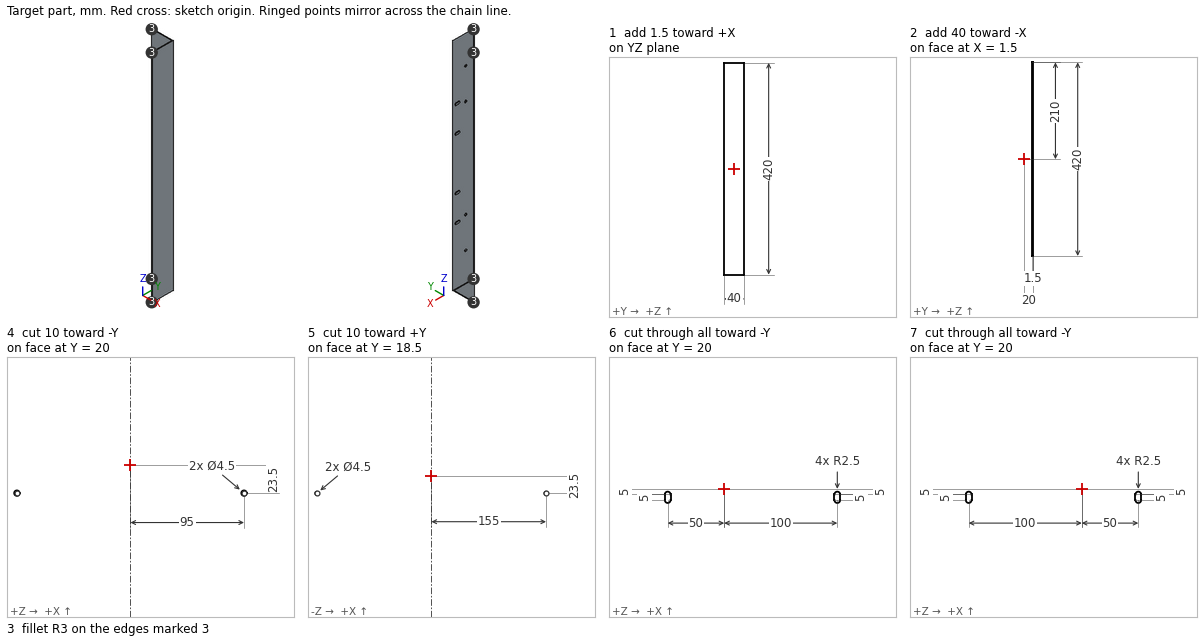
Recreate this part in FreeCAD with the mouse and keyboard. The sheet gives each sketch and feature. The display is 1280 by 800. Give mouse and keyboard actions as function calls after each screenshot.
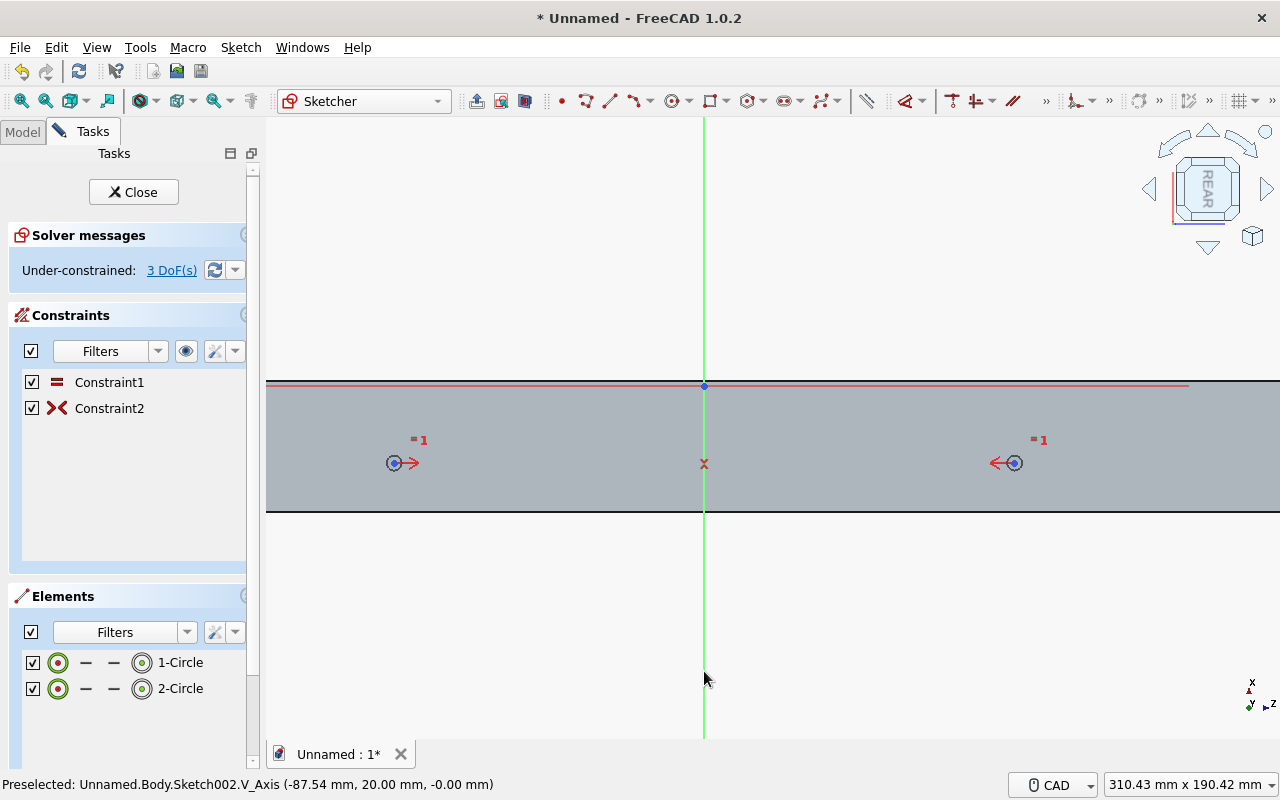
scroll(1020, 468, up, 5)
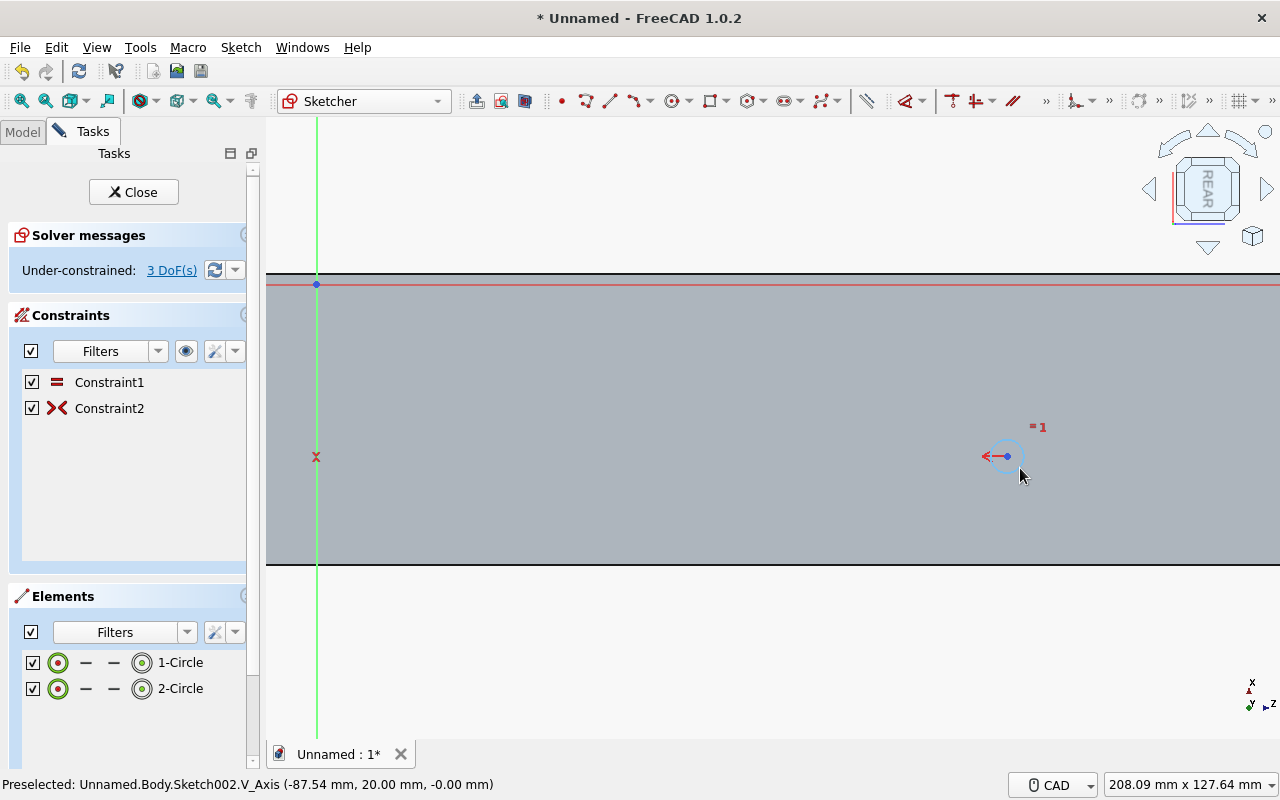
click(1018, 468)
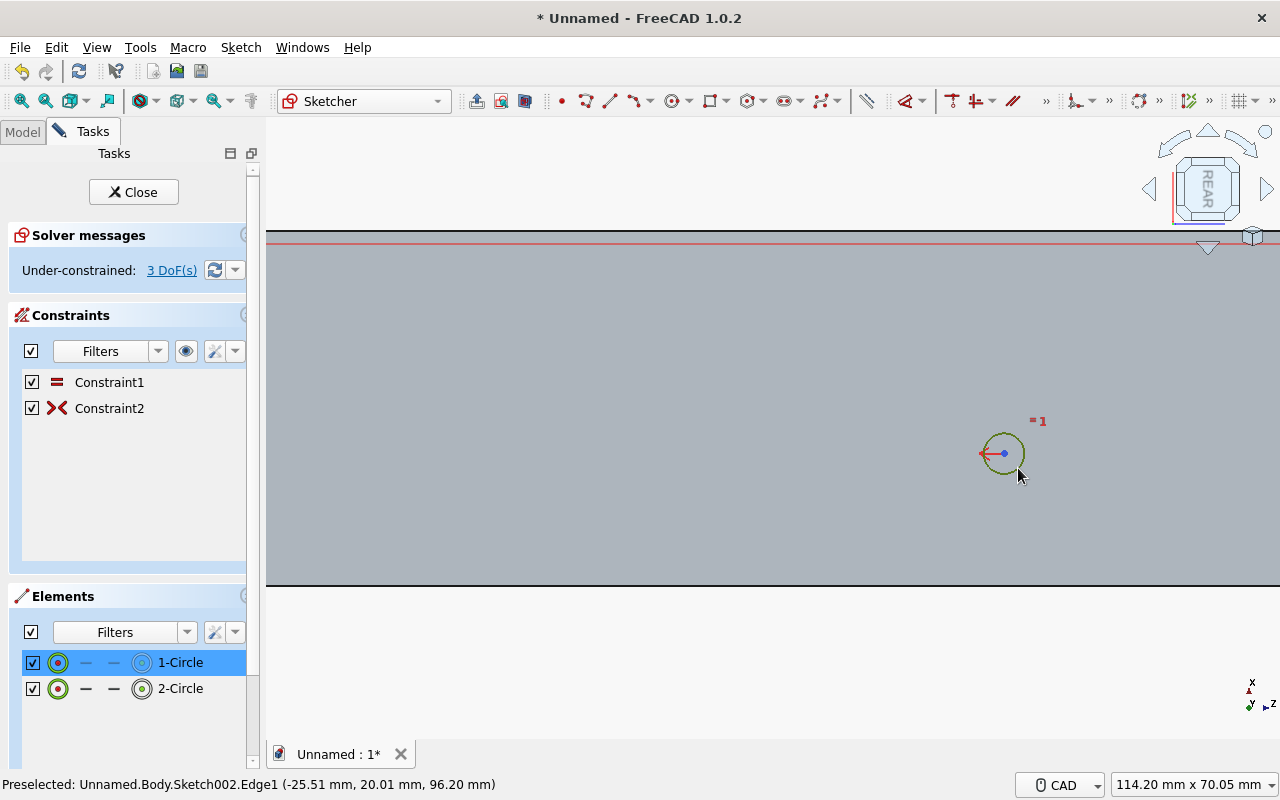
click(924, 102)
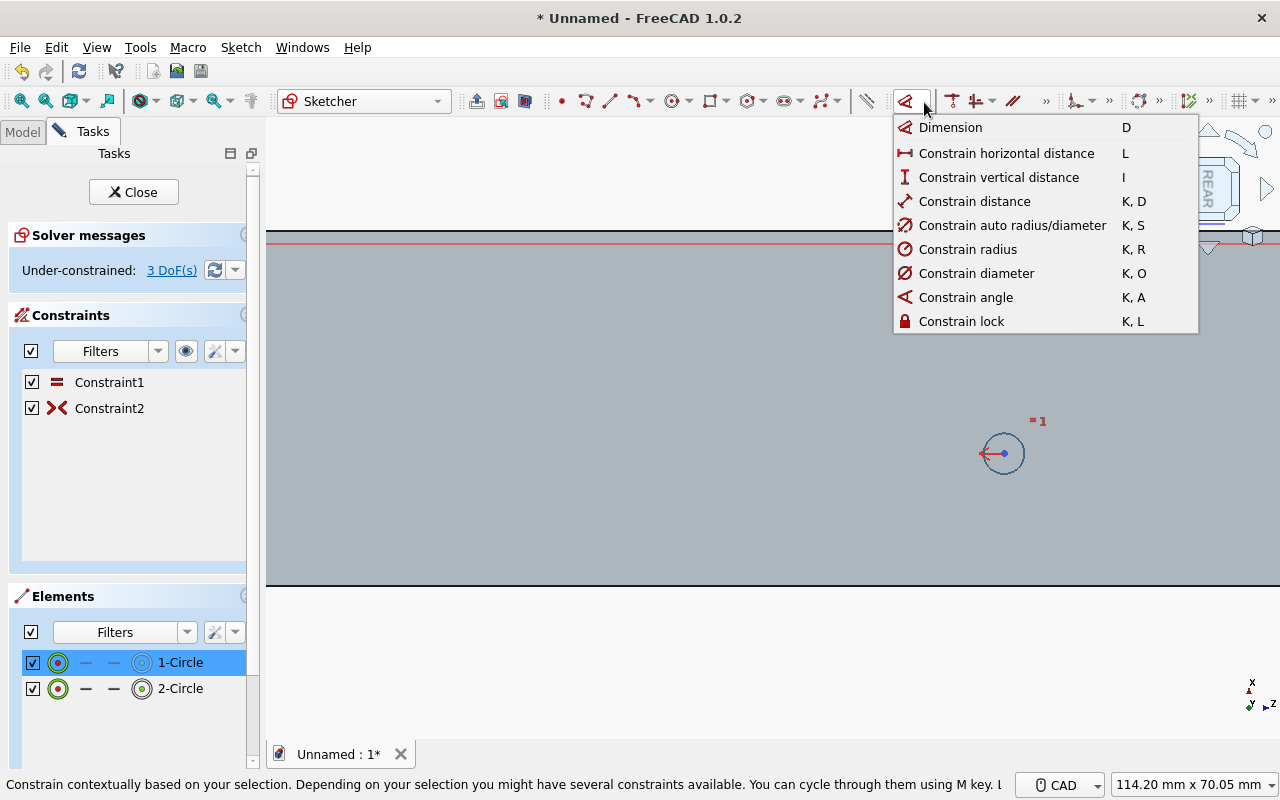
click(1046, 273)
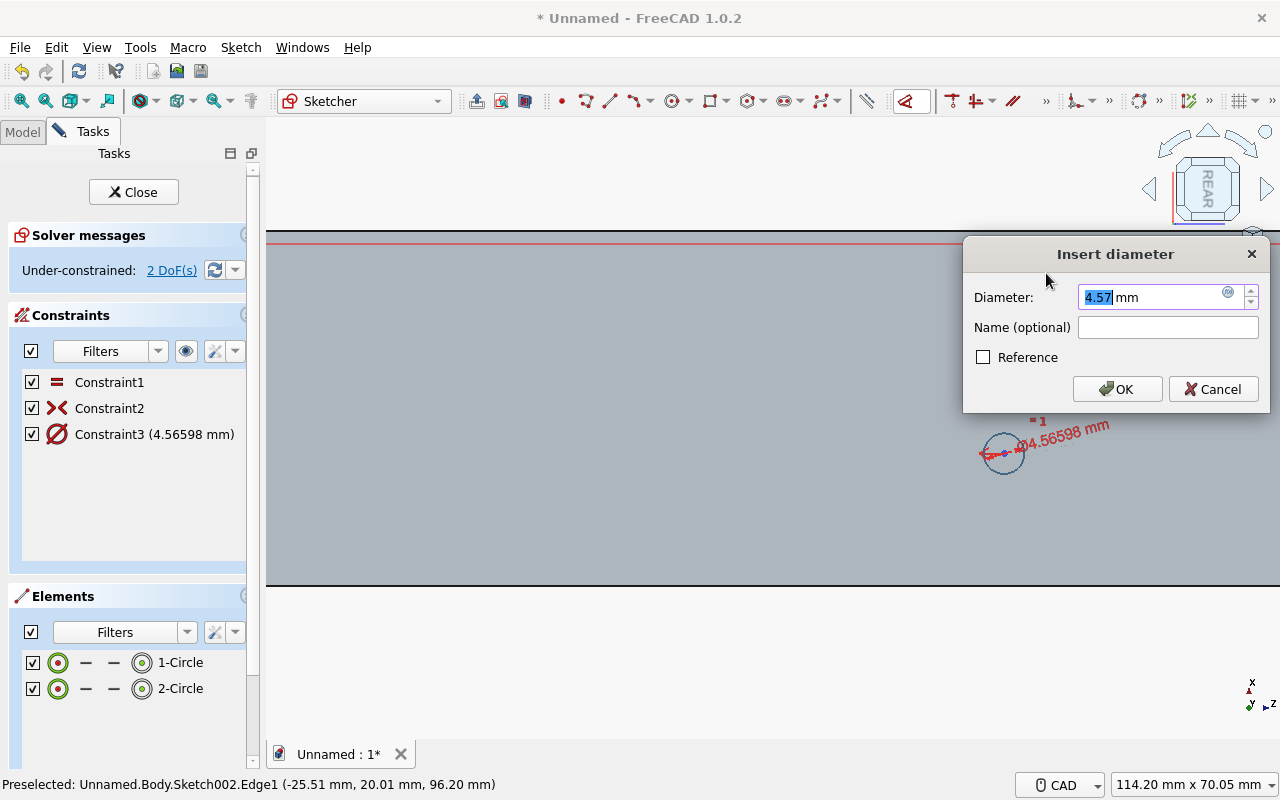
text(4.5)
key(Return)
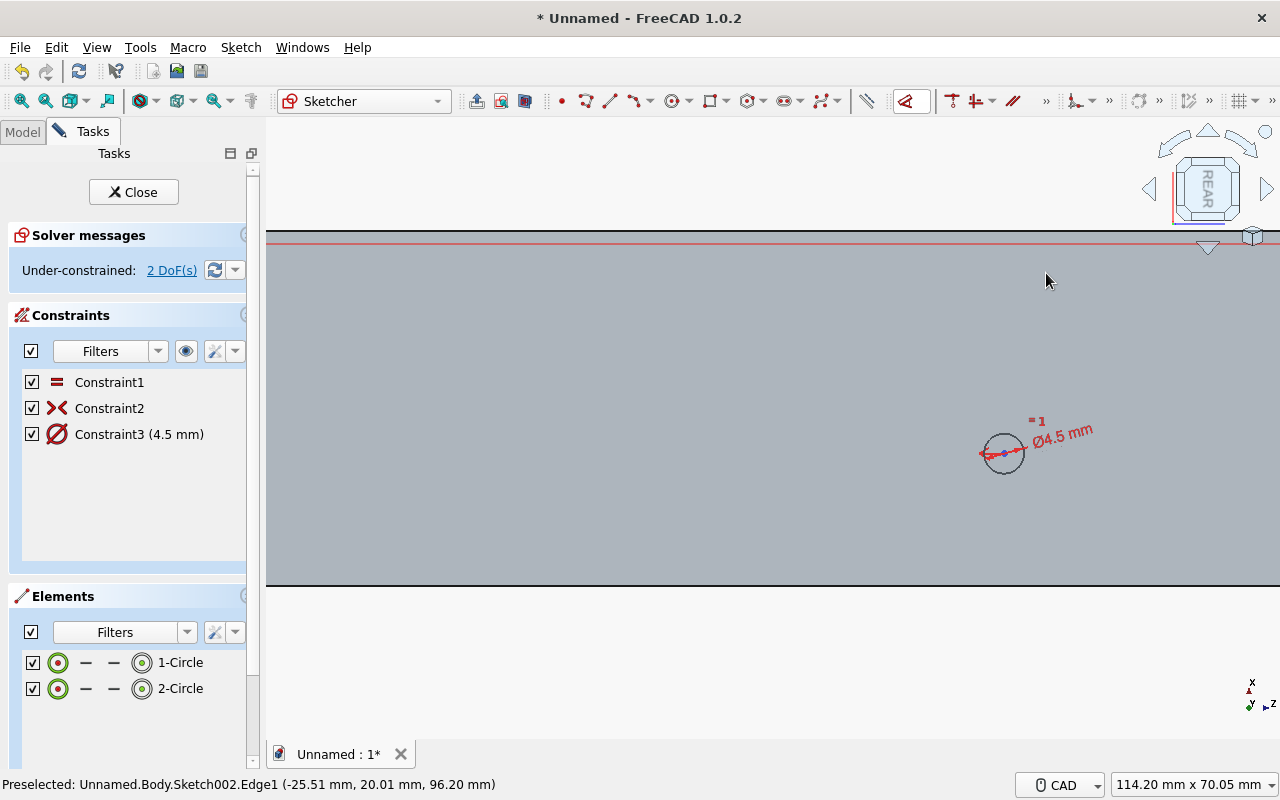
click(1004, 454)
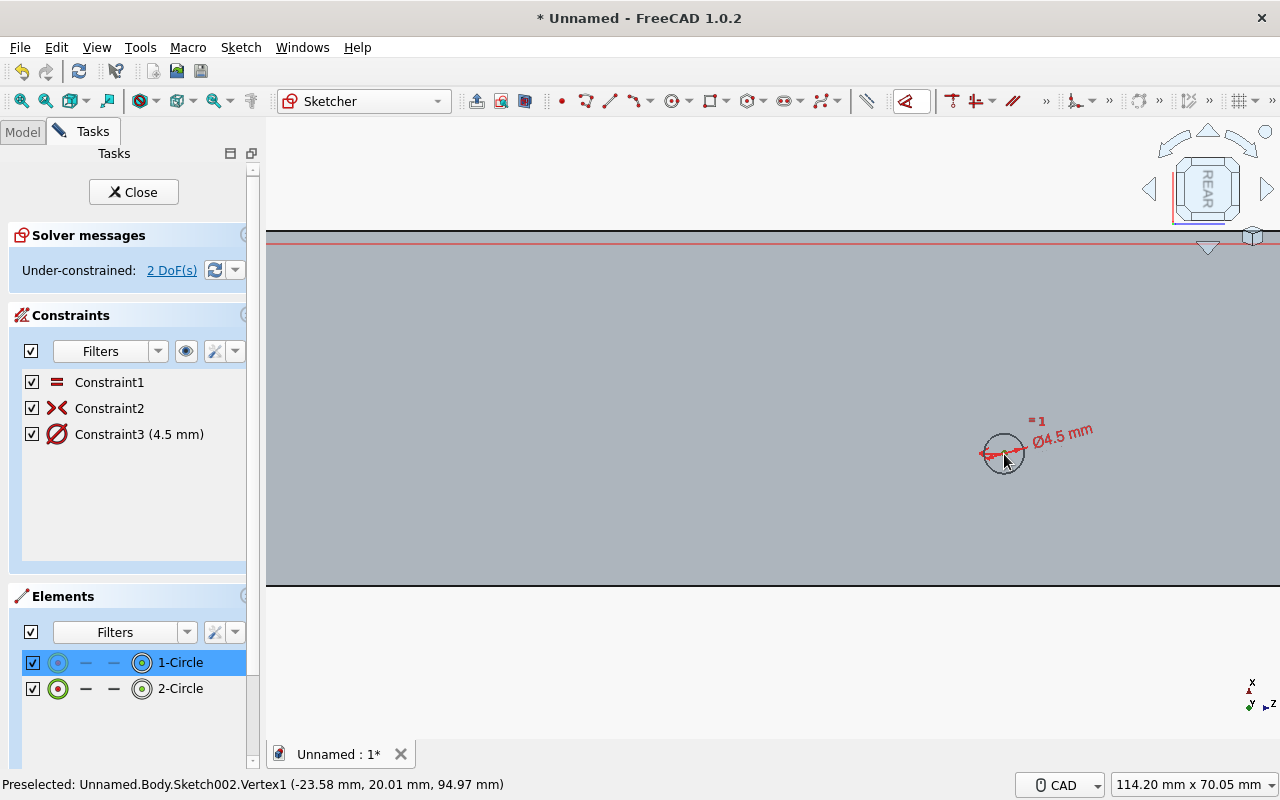
click(924, 102)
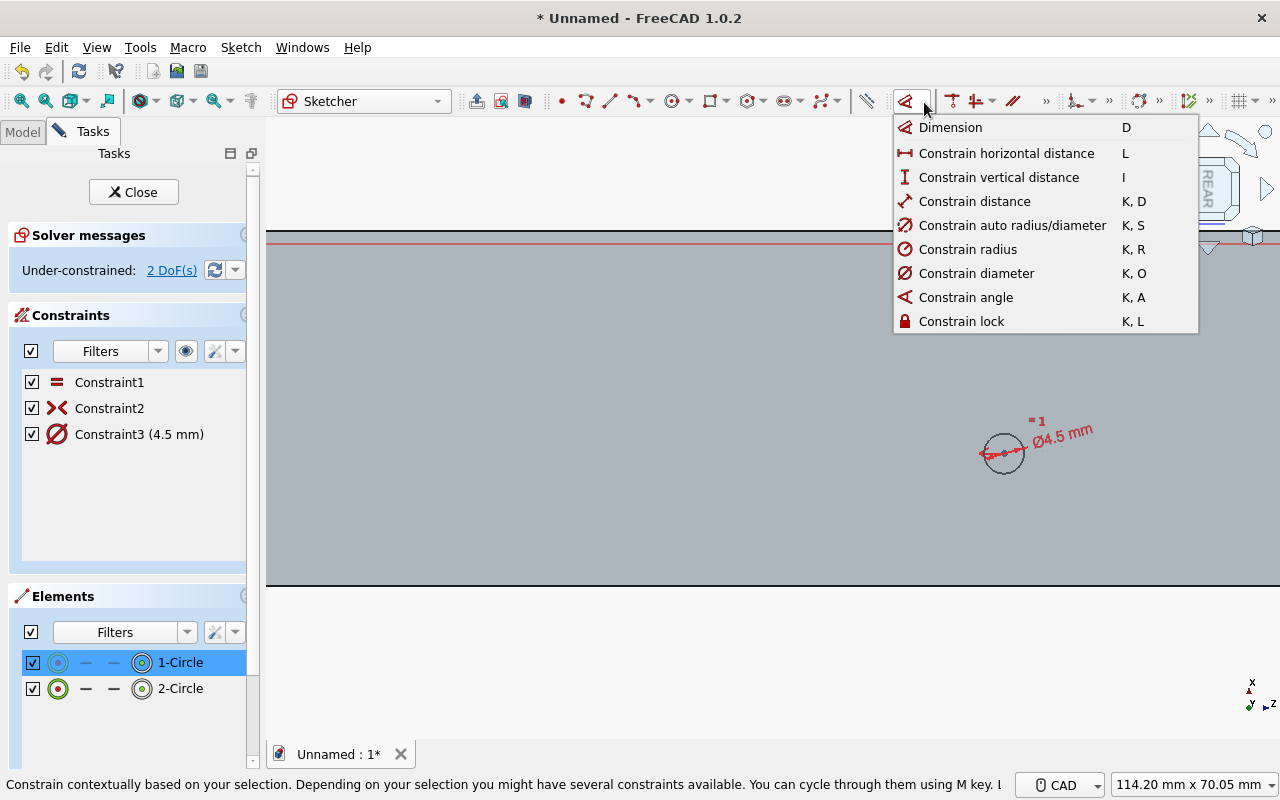
click(1046, 153)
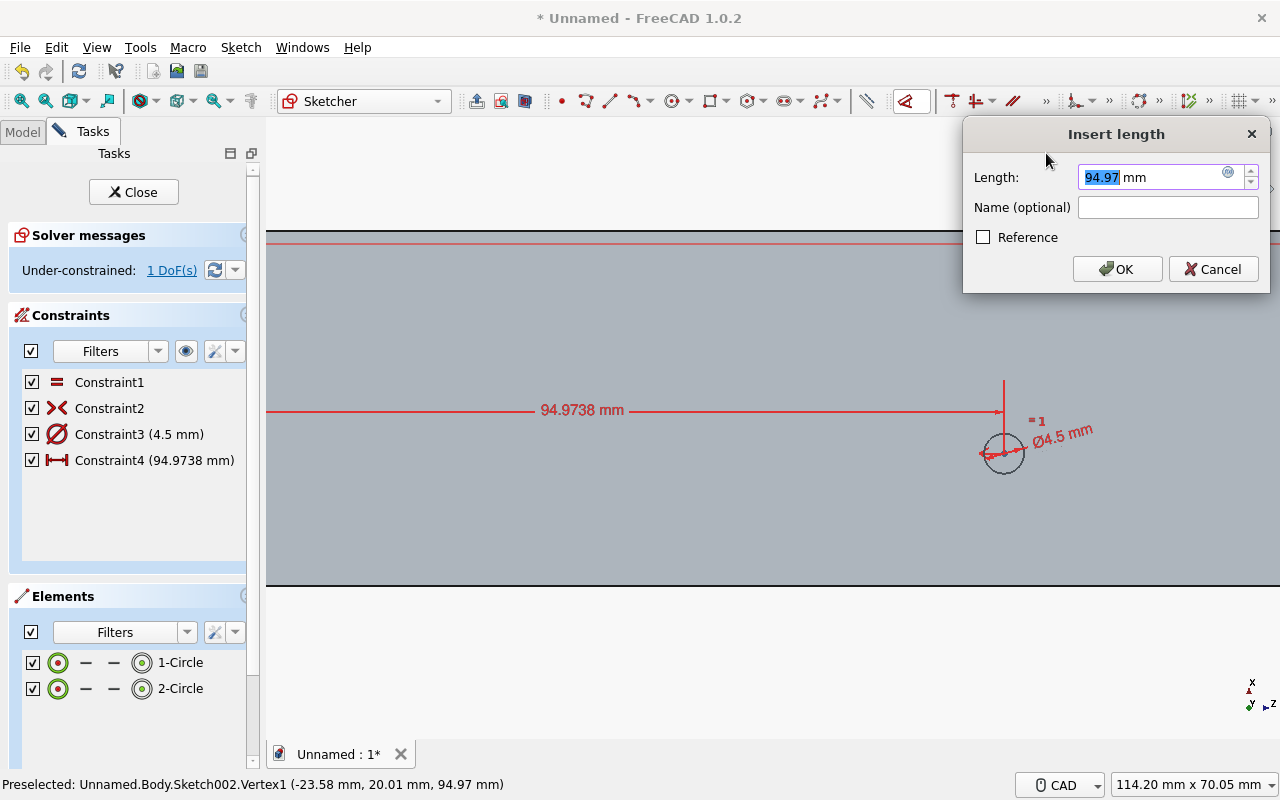
text(95)
key(Return)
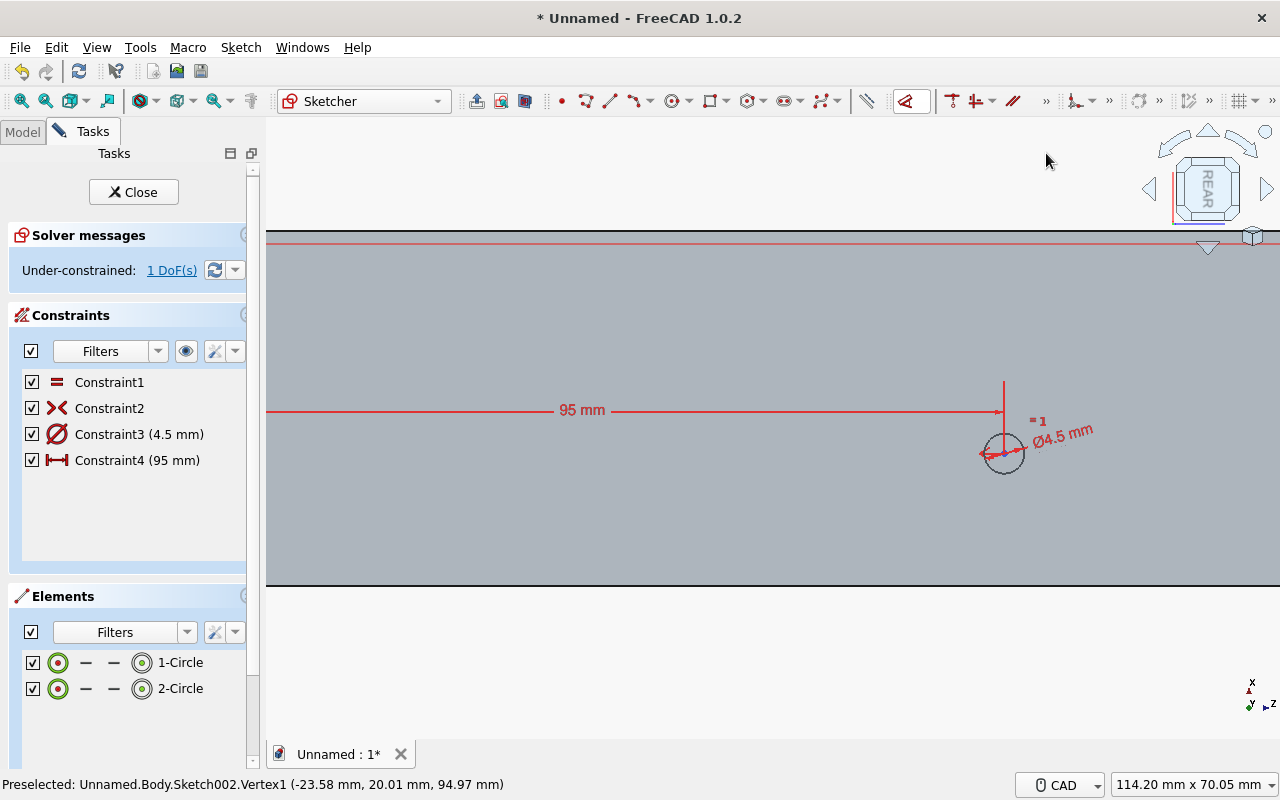
click(1004, 454)